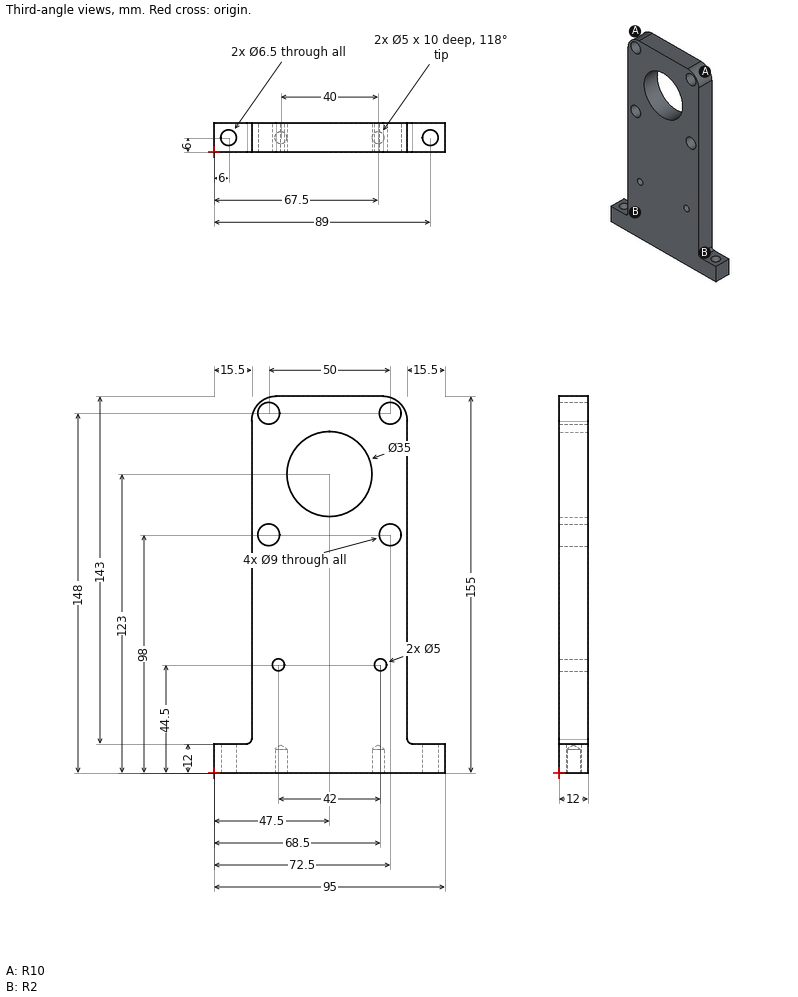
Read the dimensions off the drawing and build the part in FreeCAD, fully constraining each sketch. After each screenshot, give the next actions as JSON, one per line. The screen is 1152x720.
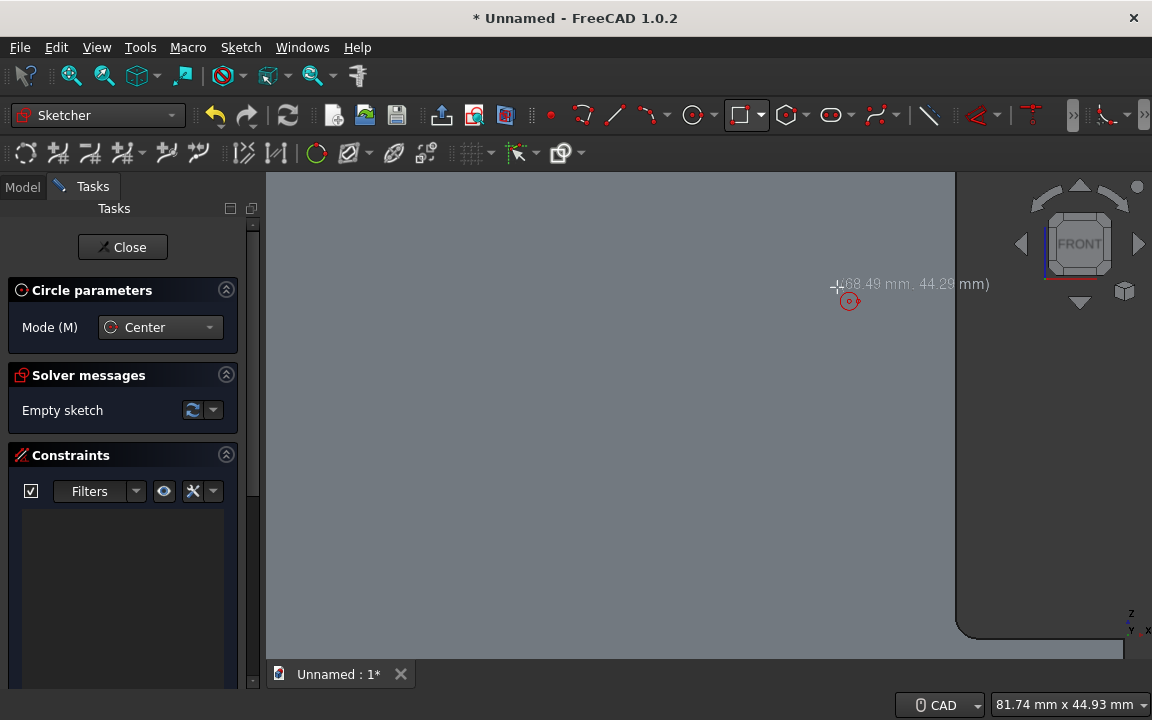
{"action": "left_click", "coordinate": [837, 286]}
{"action": "left_click", "coordinate": [856, 267]}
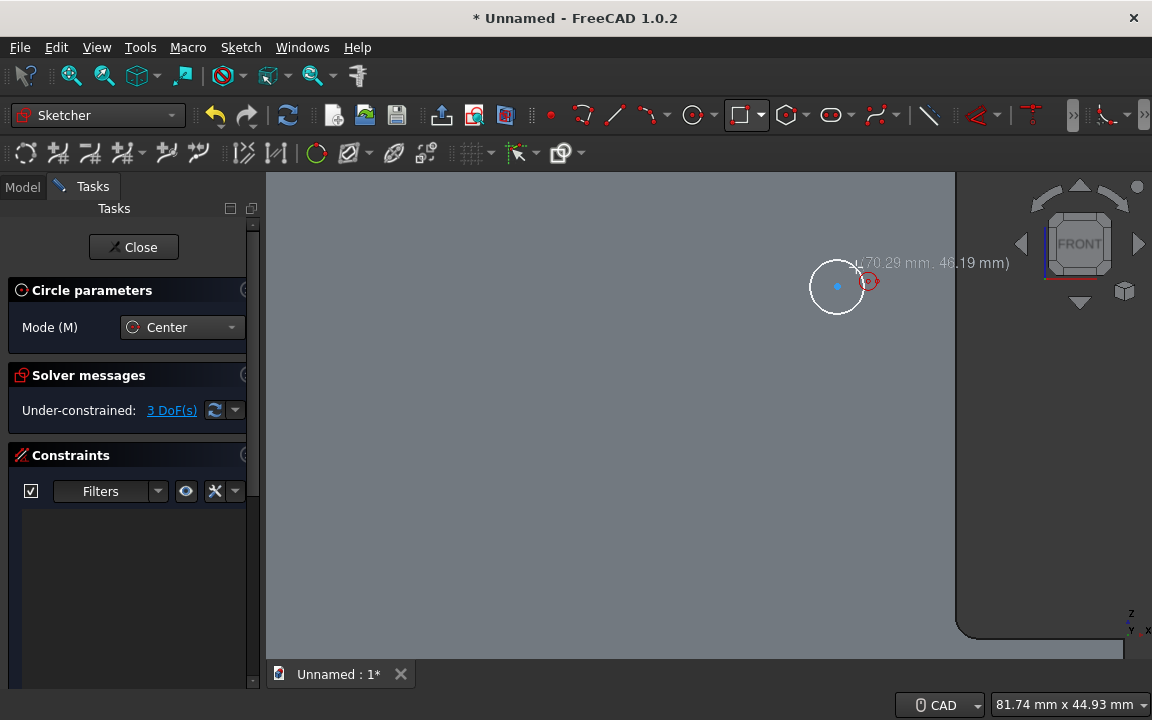
{"action": "left_click", "coordinate": [381, 286]}
{"action": "left_click", "coordinate": [401, 267]}
{"action": "key", "text": "Escape"}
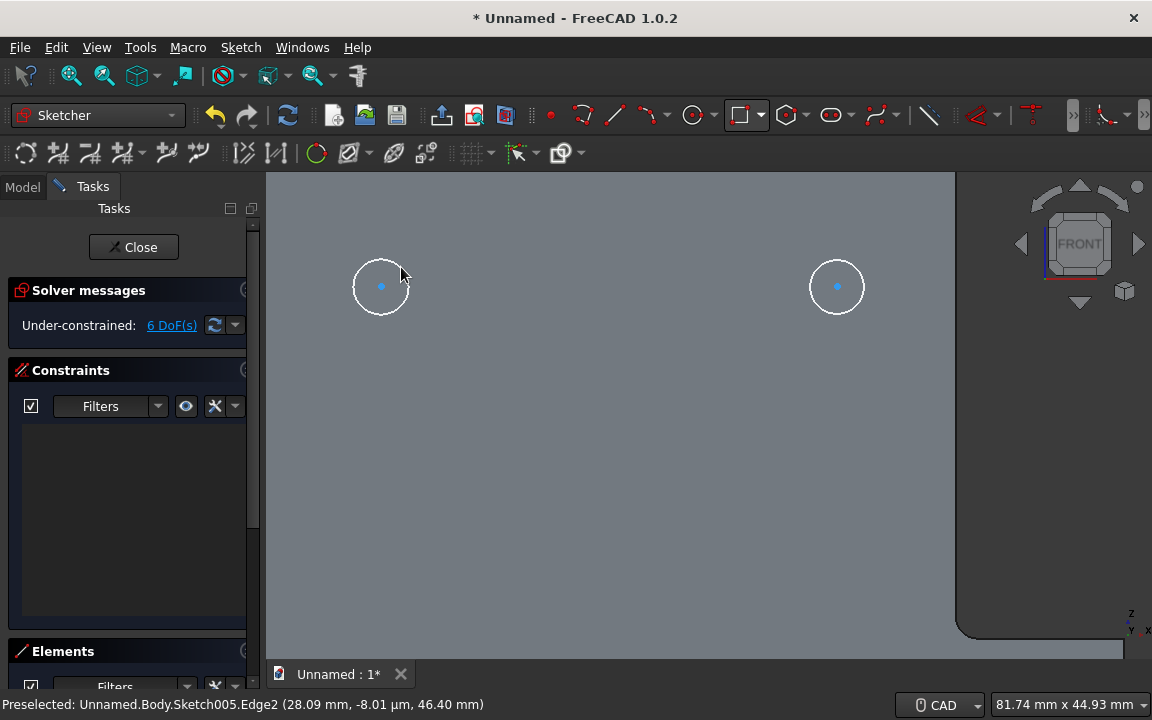
{"action": "left_click", "coordinate": [856, 268]}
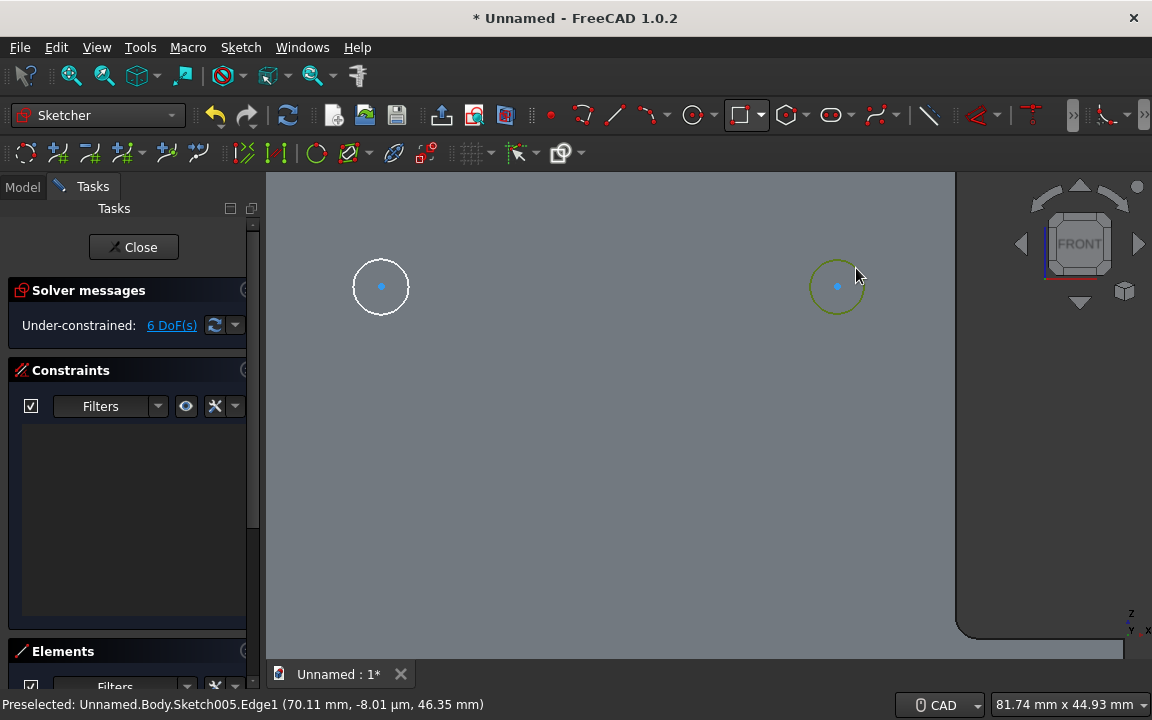
{"action": "left_click", "coordinate": [400, 267]}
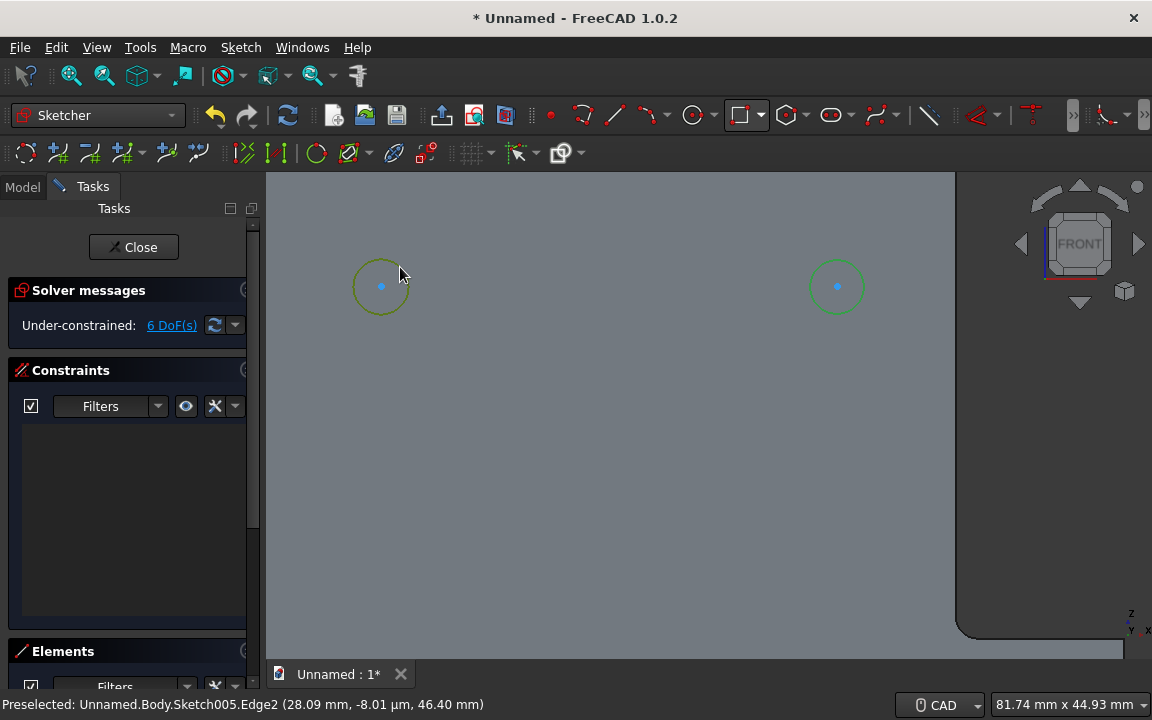
{"action": "key", "text": "e"}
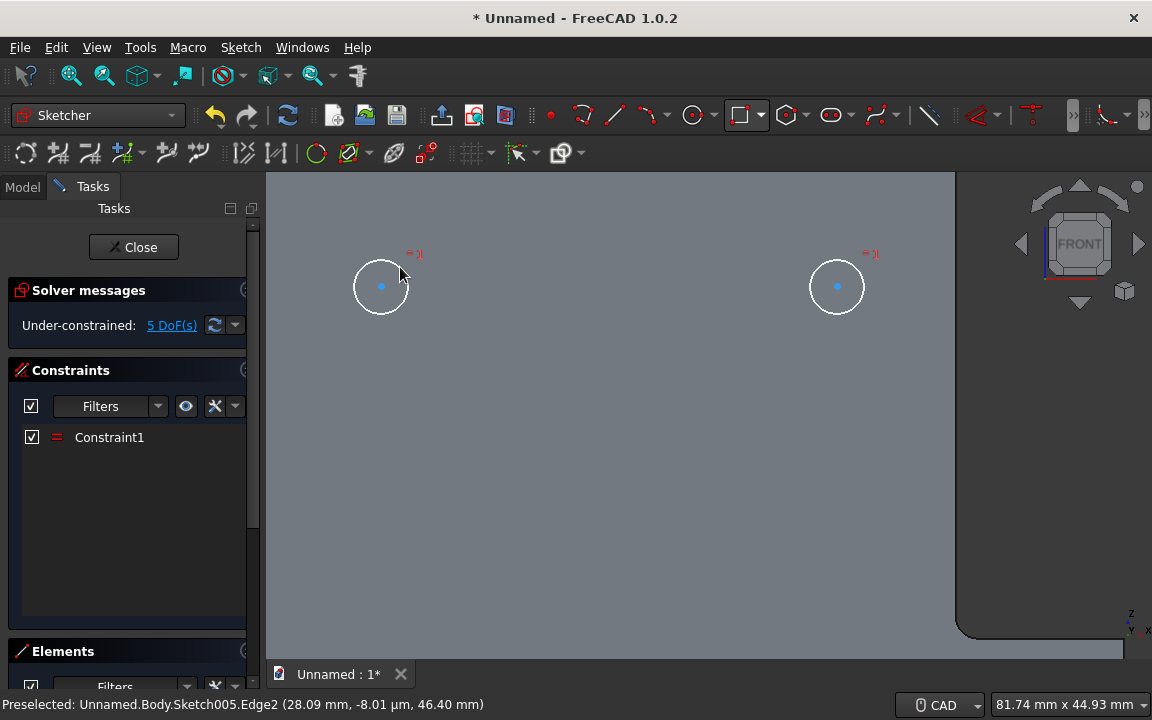
{"action": "left_click", "coordinate": [837, 287]}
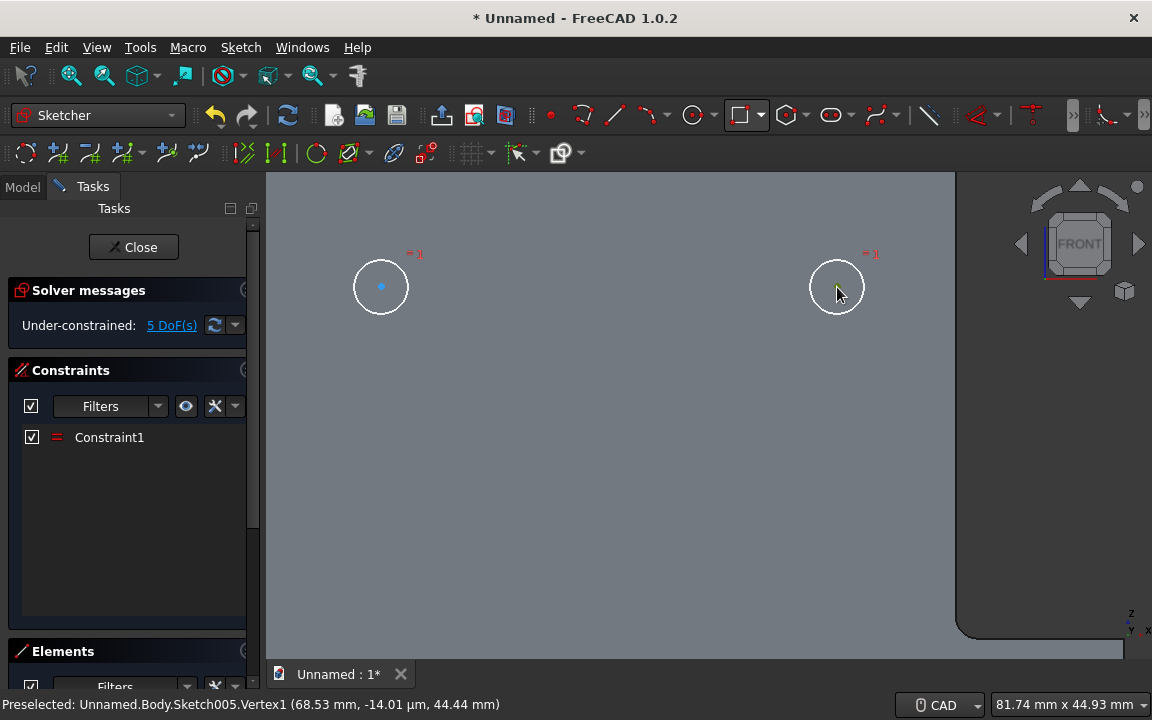
{"action": "left_click", "coordinate": [381, 287]}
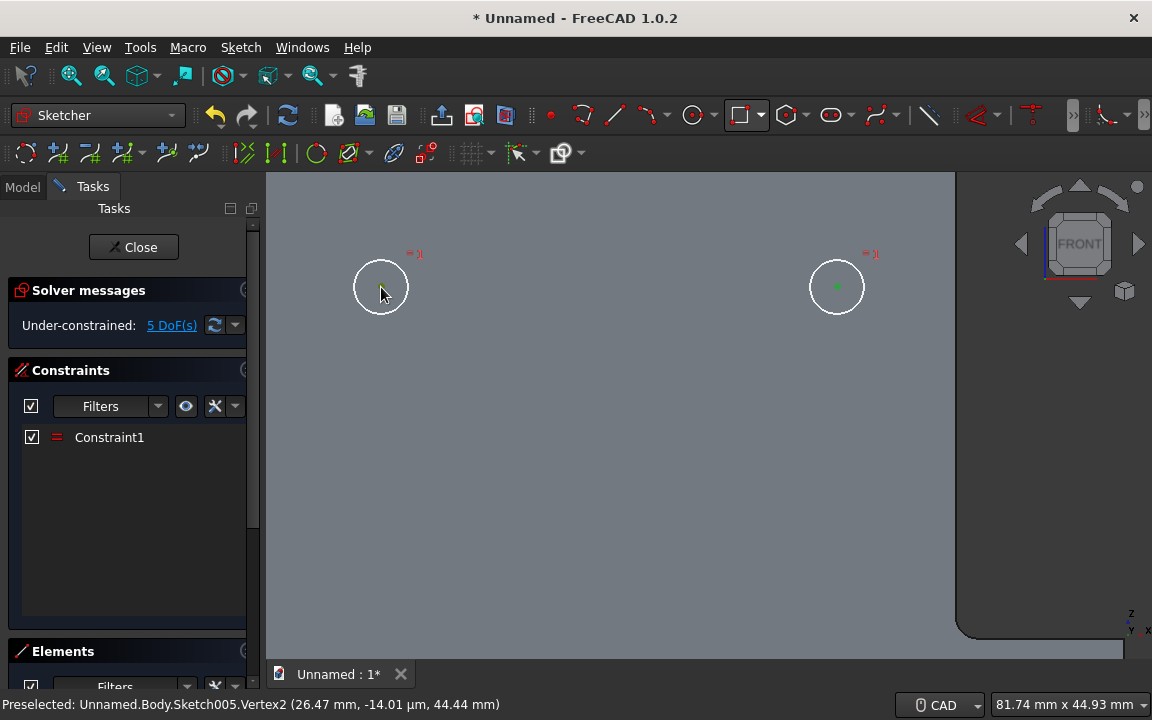
{"action": "key", "text": "h"}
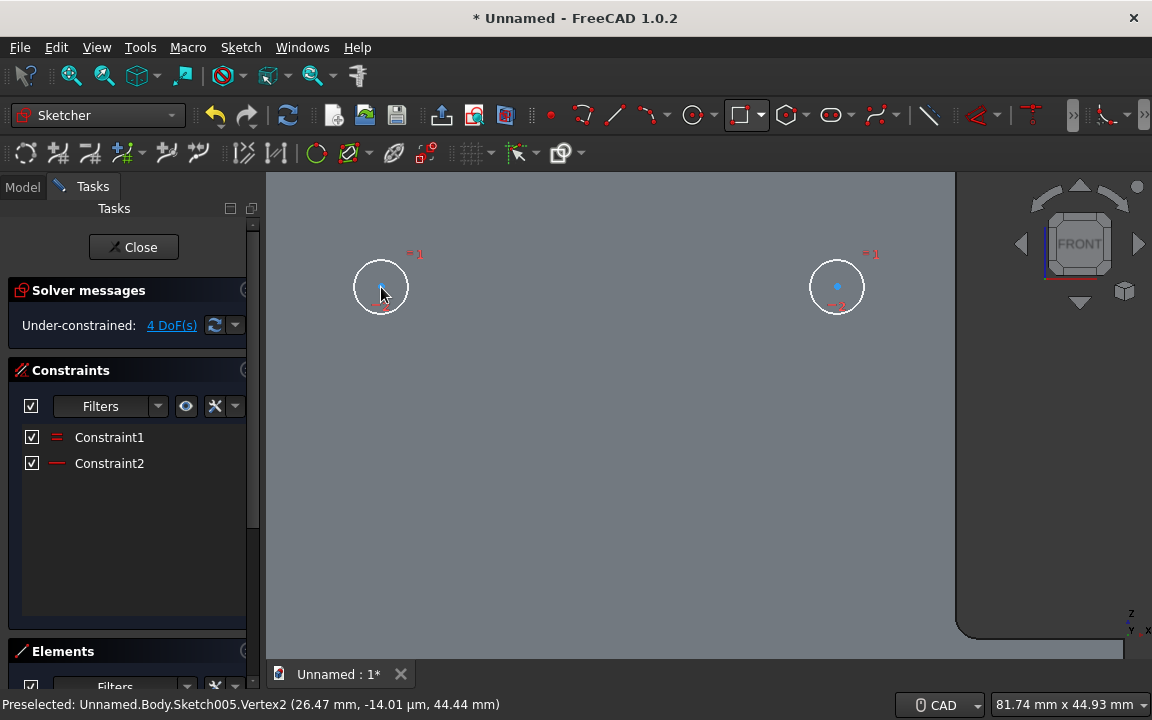
{"action": "left_click", "coordinate": [976, 116]}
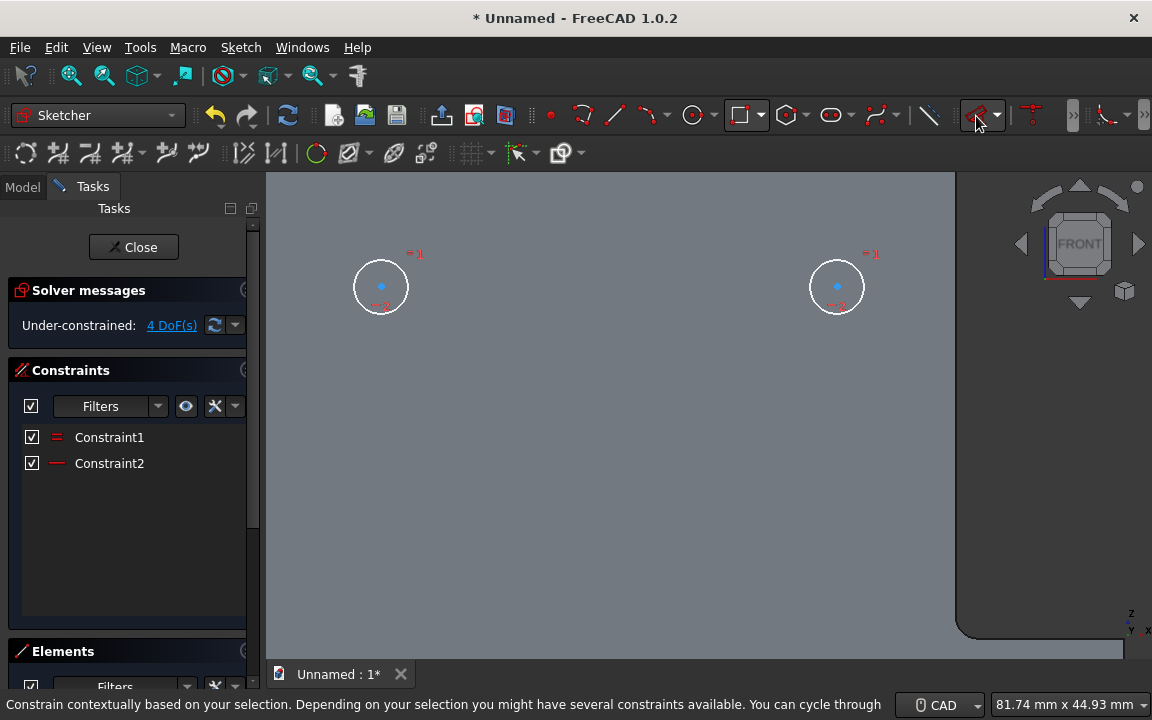
{"action": "left_click", "coordinate": [856, 268]}
{"action": "left_click", "coordinate": [879, 245]}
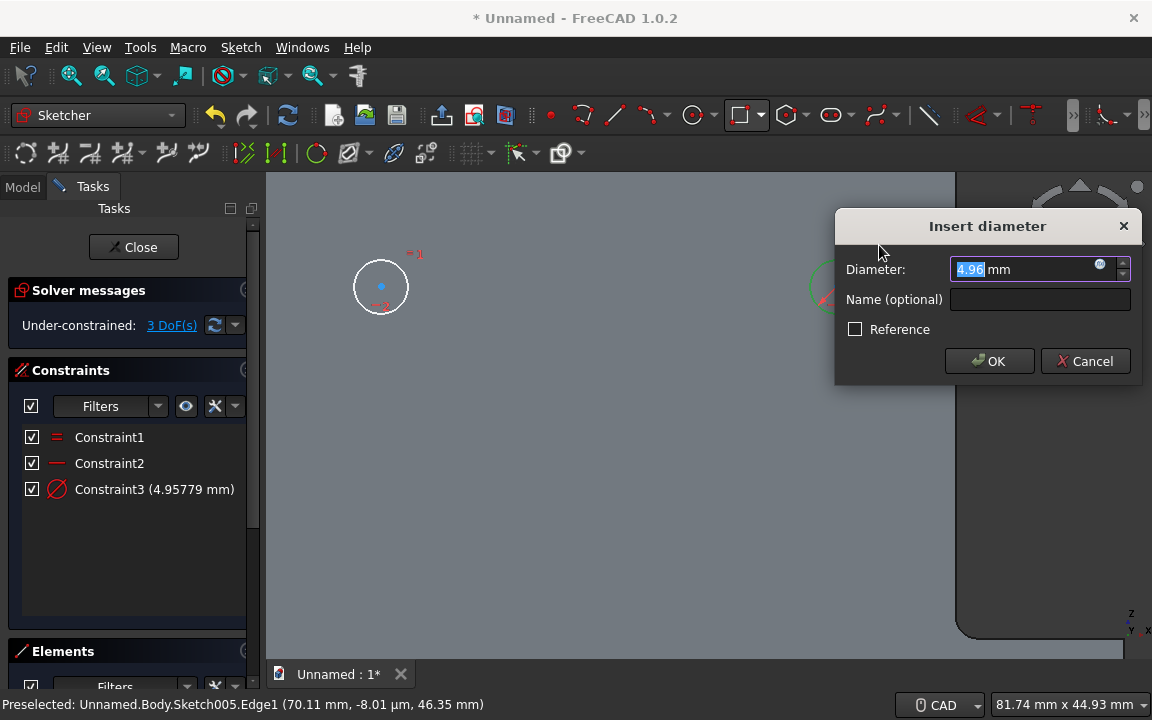
{"action": "type", "text": "5"}
{"action": "key", "text": "Return"}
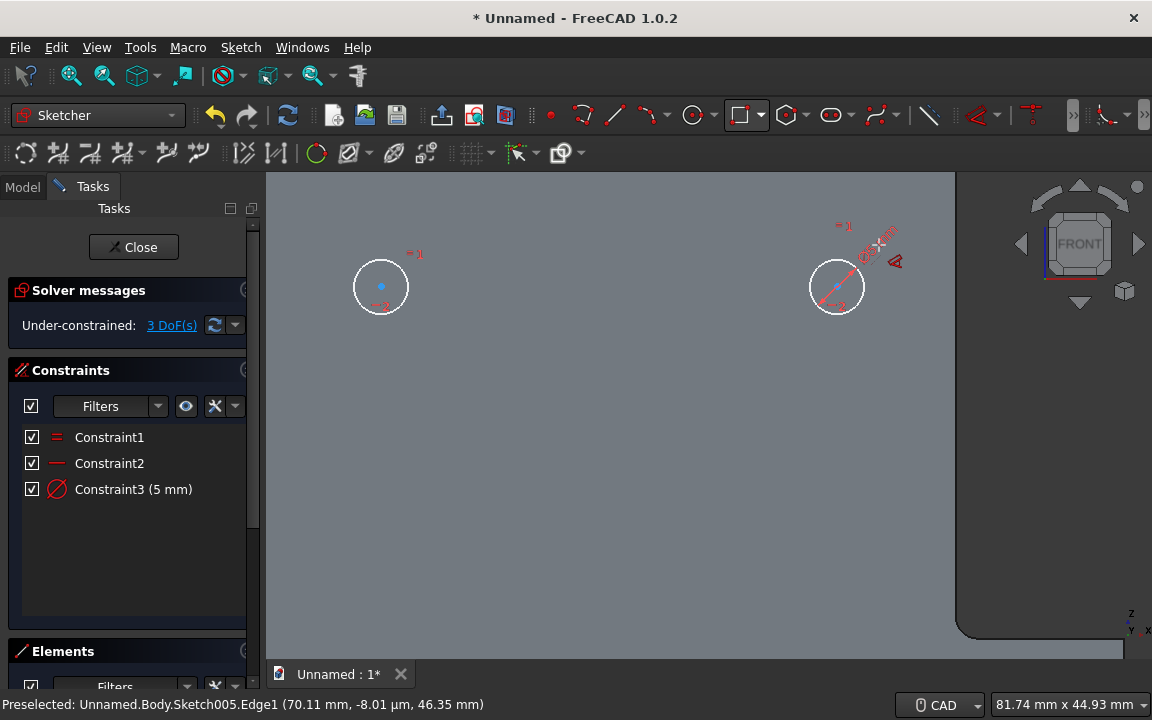
{"action": "left_click", "coordinate": [837, 287]}